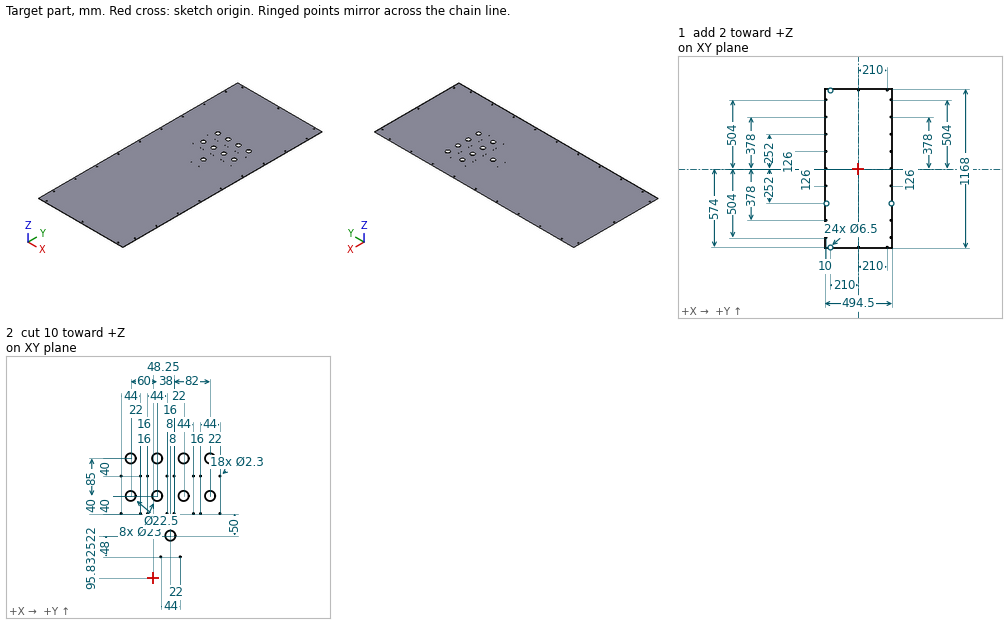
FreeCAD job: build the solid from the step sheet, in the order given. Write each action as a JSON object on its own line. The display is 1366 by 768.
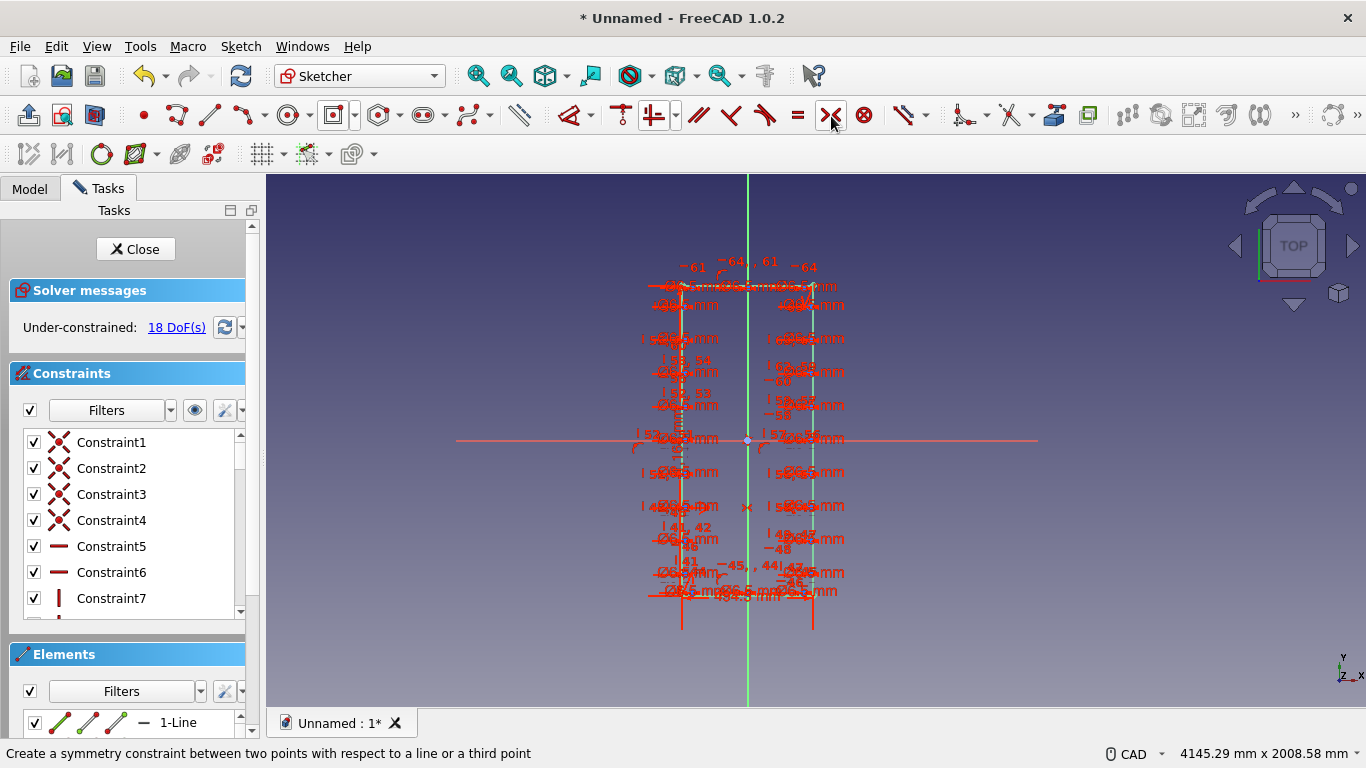
{"action": "left_click", "coordinate": [692, 593]}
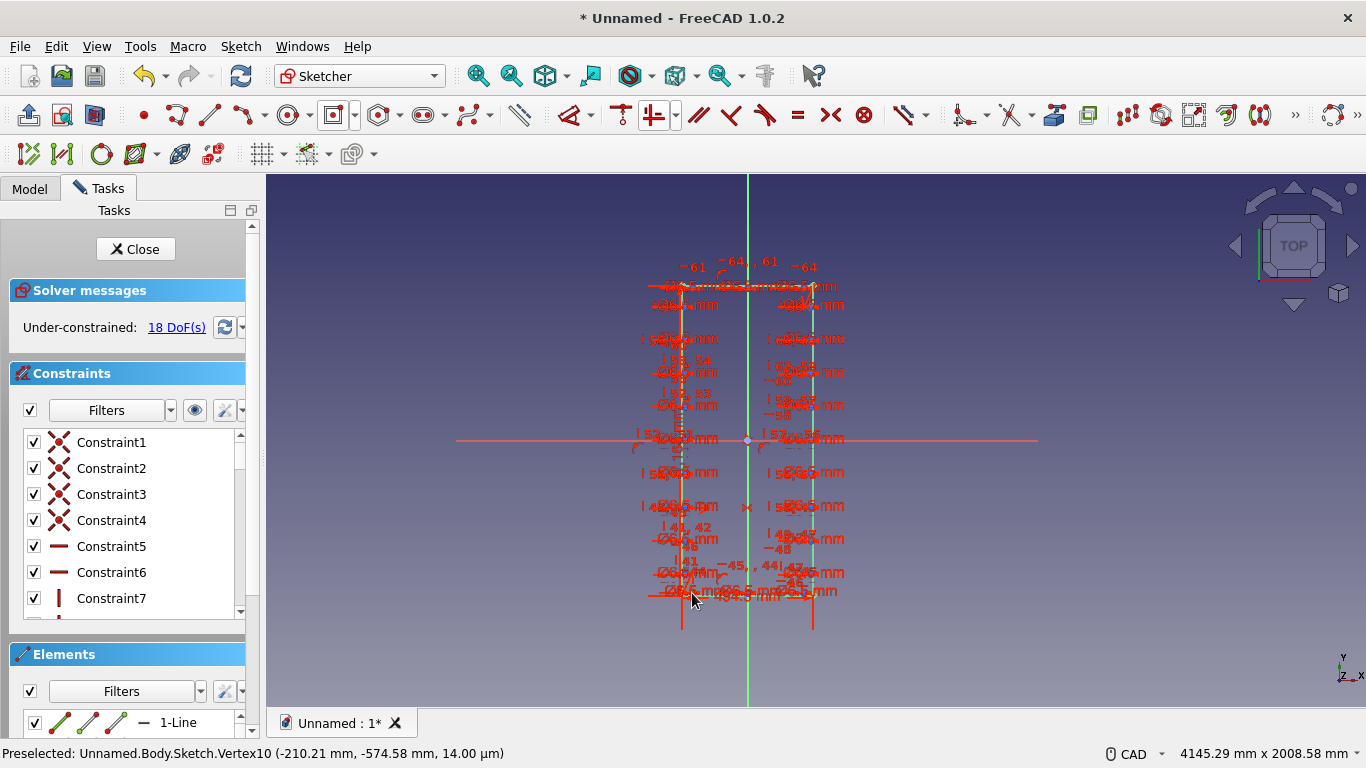
{"action": "left_click", "coordinate": [692, 288]}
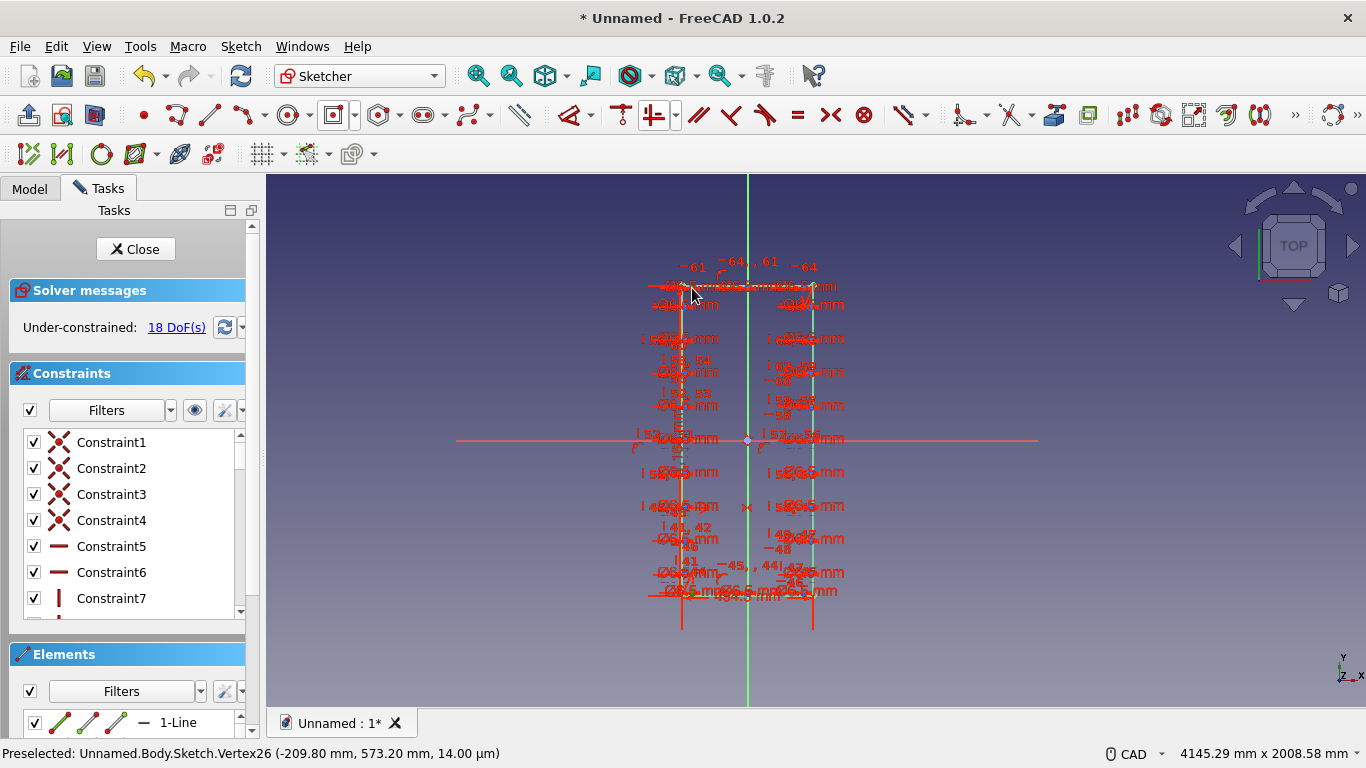
{"action": "left_click", "coordinate": [488, 441]}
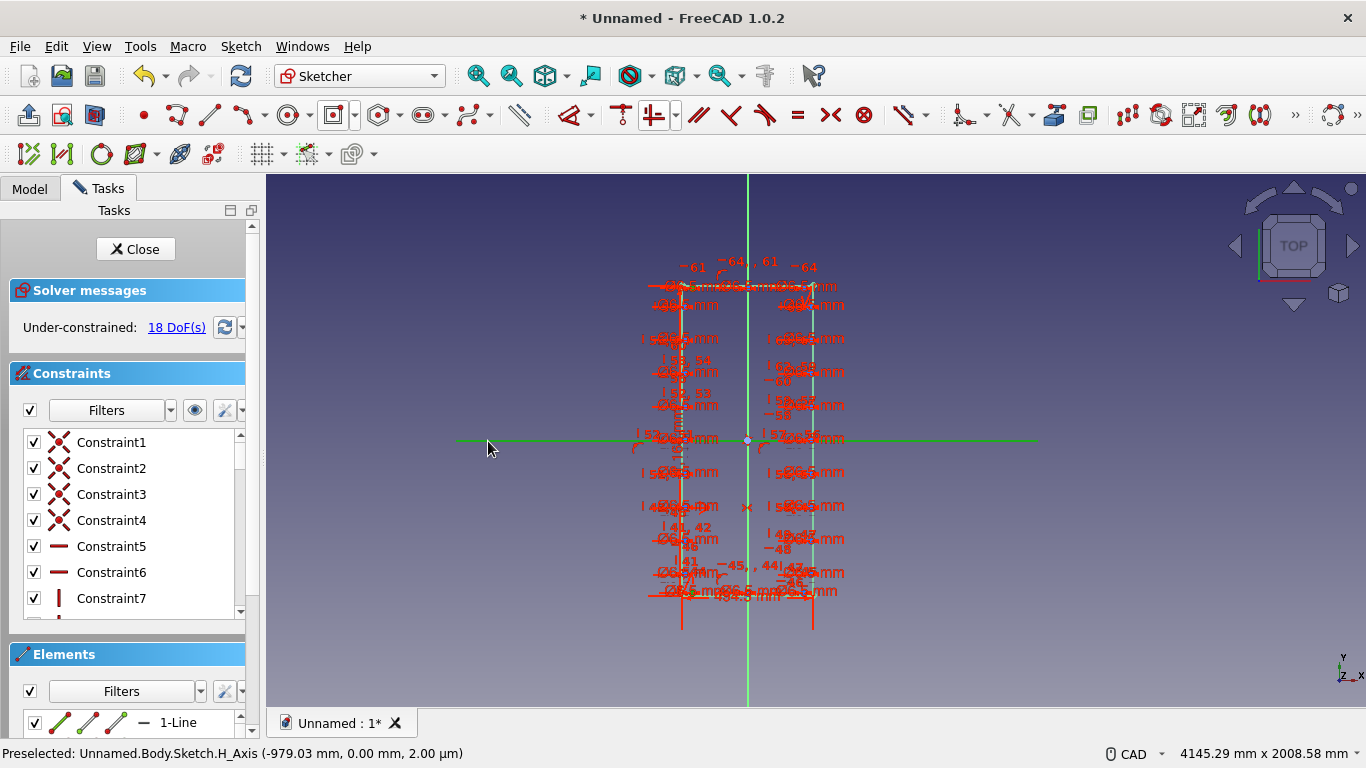
{"action": "left_click", "coordinate": [831, 116]}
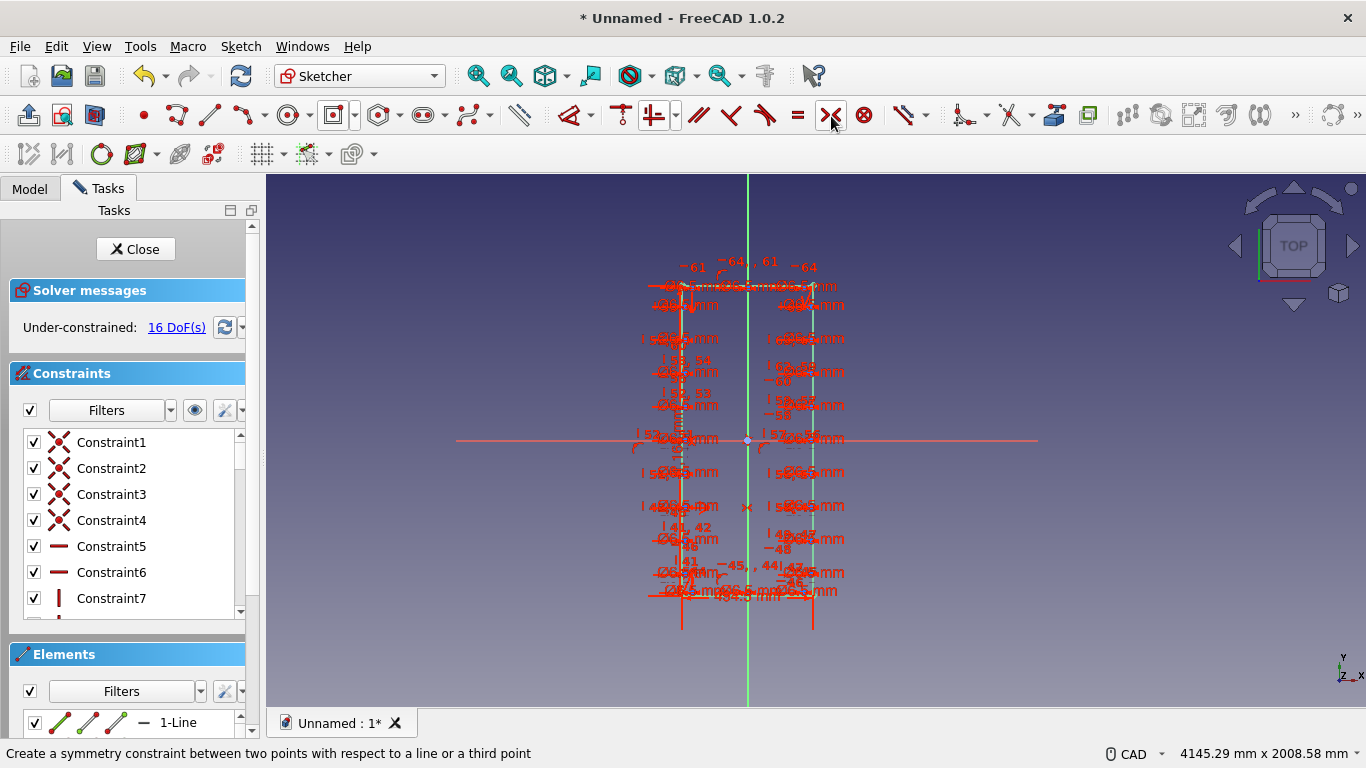
{"action": "left_click", "coordinate": [568, 116]}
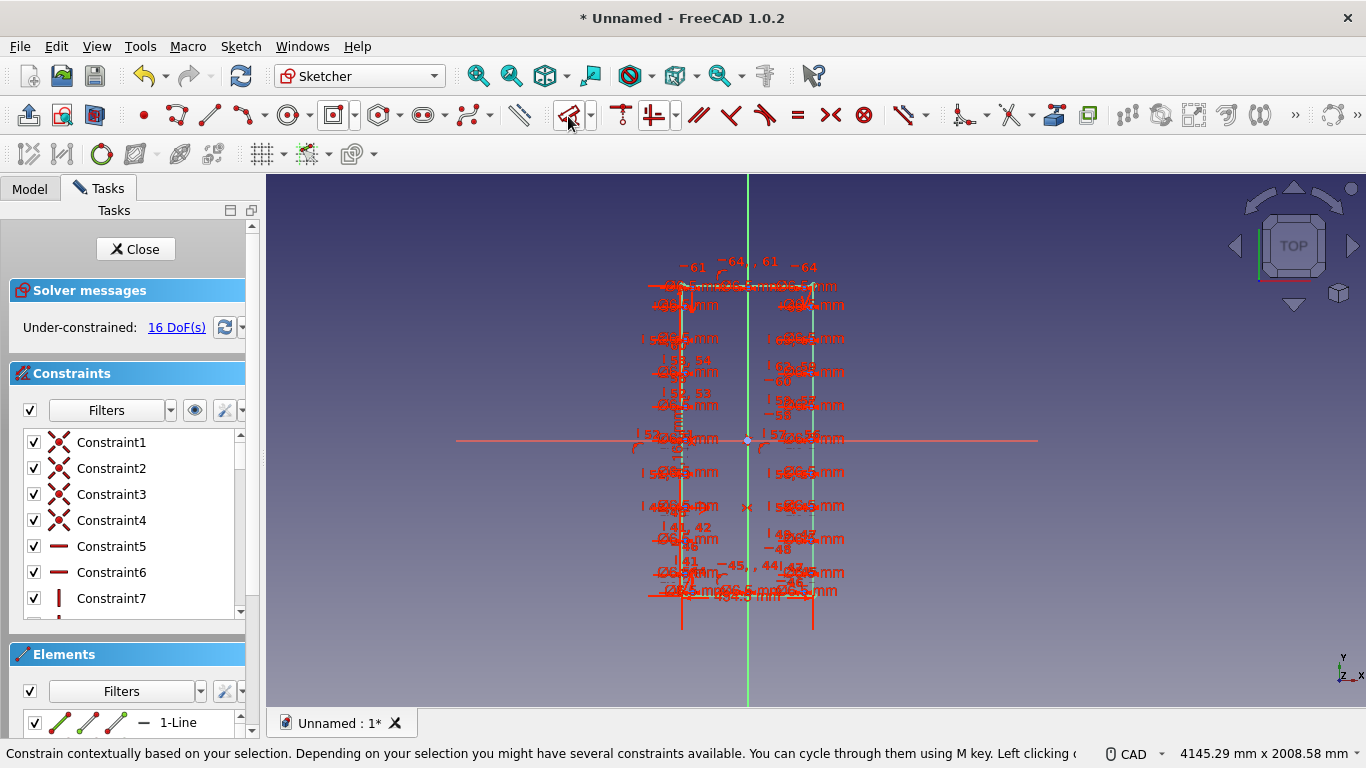
{"action": "left_click", "coordinate": [692, 593]}
{"action": "left_click", "coordinate": [720, 627]}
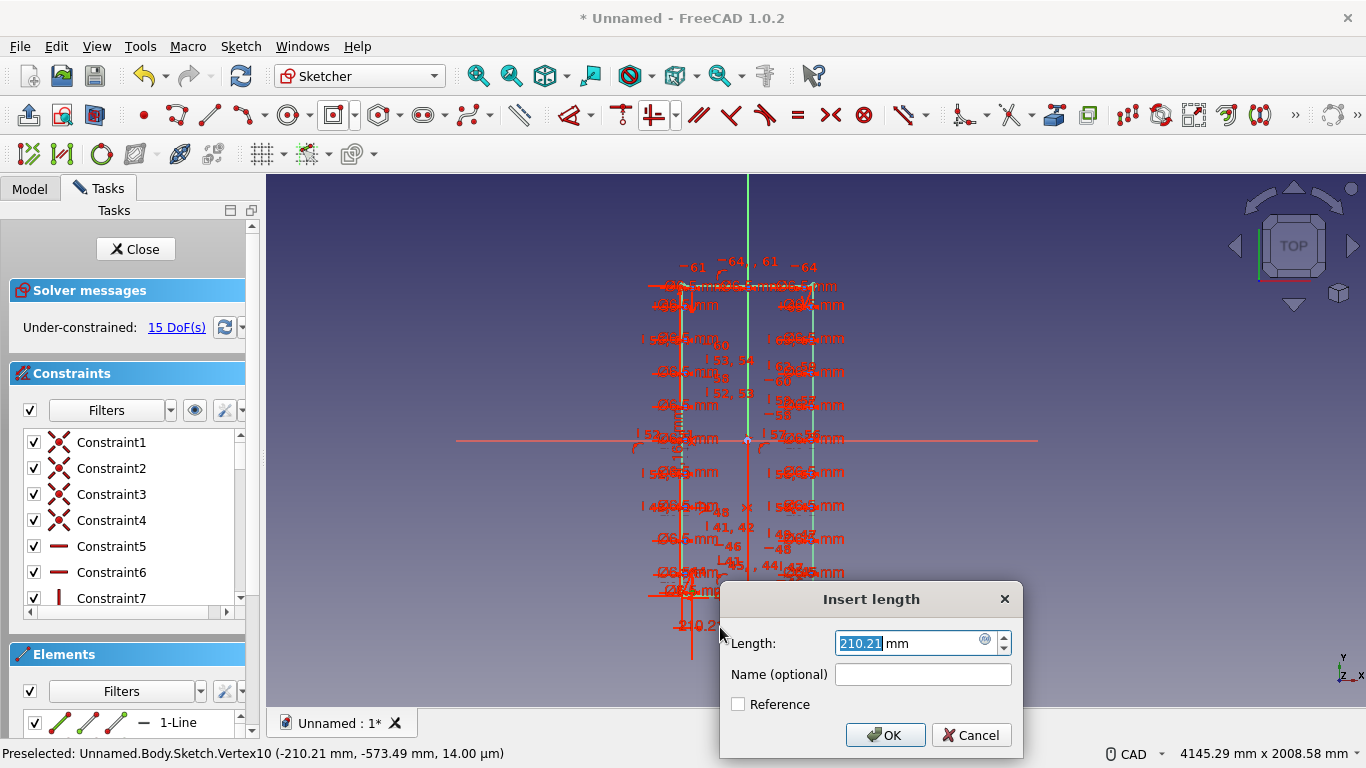
{"action": "type", "text": "210"}
{"action": "key", "text": "Return"}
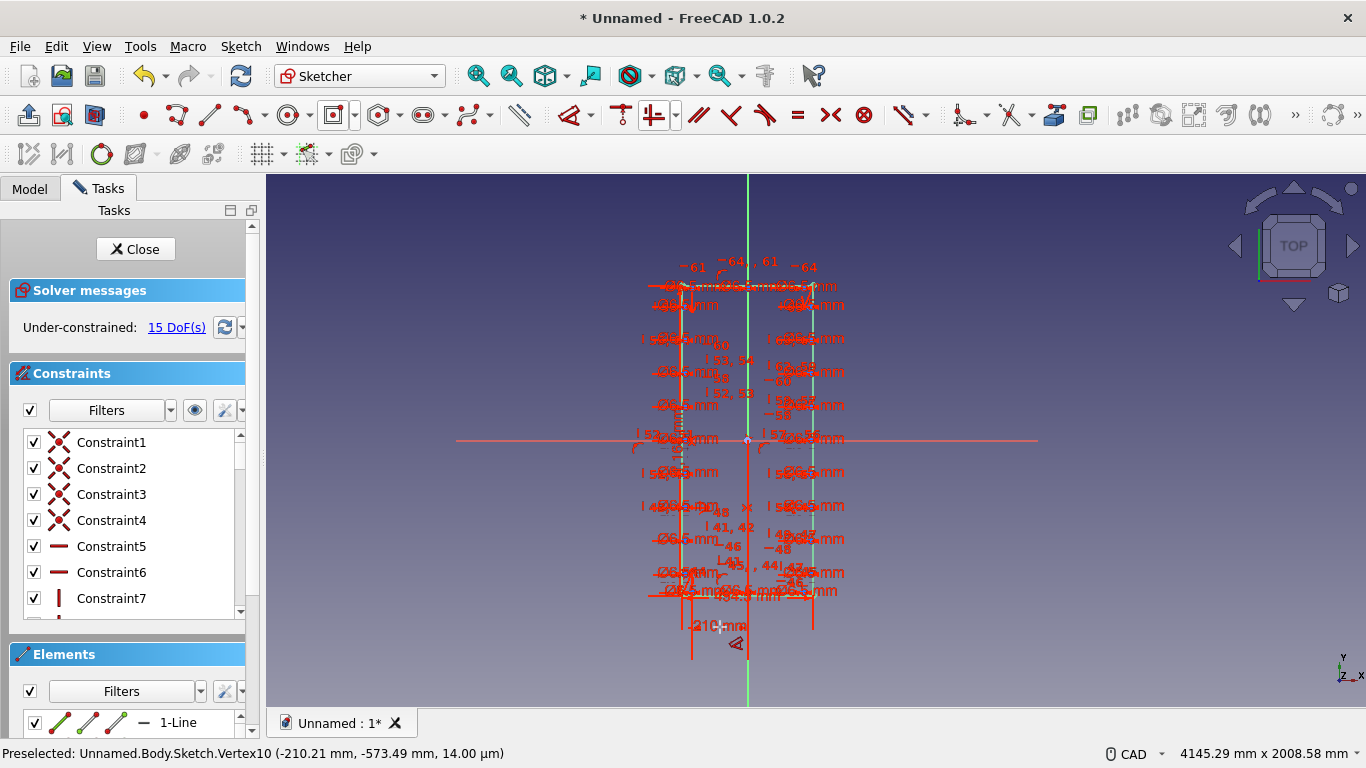
{"action": "left_click", "coordinate": [692, 593]}
{"action": "left_click", "coordinate": [658, 517]}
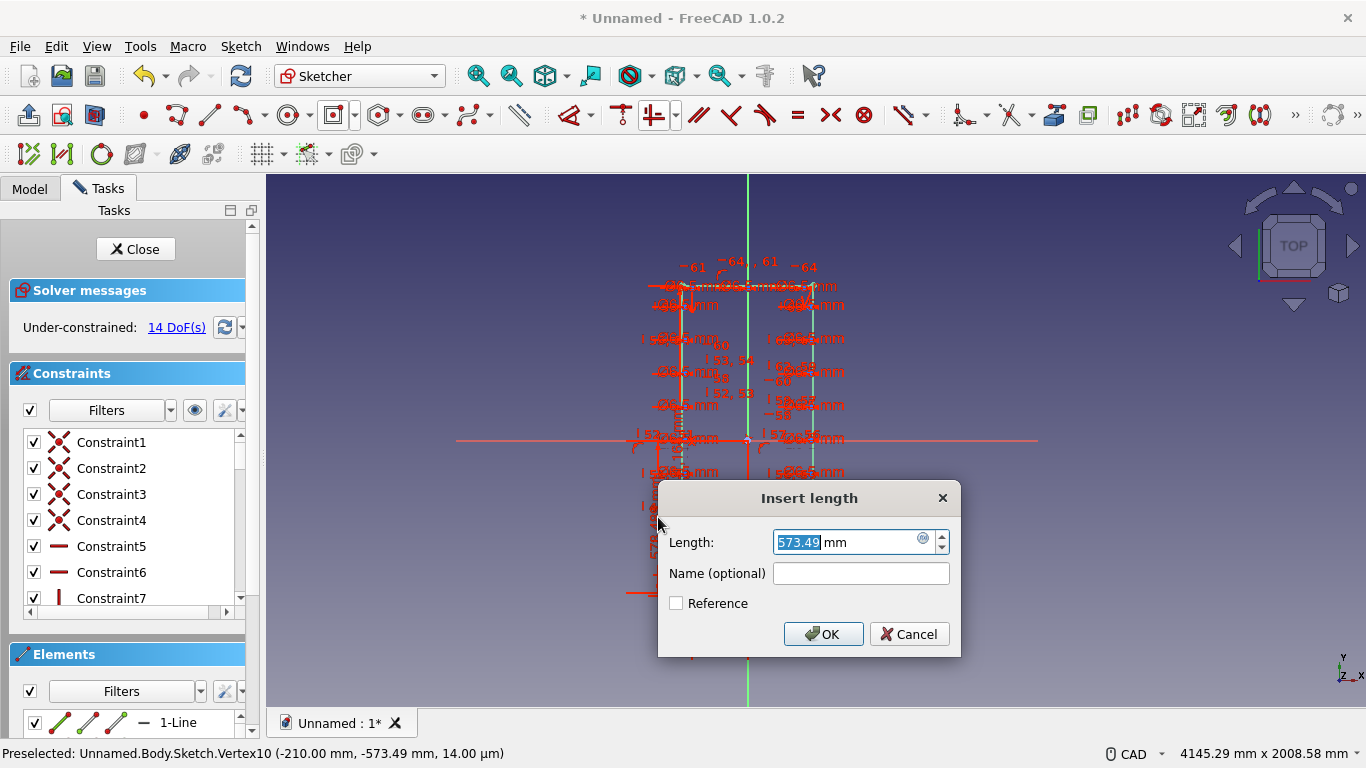
{"action": "type", "text": "574"}
{"action": "key", "text": "Return"}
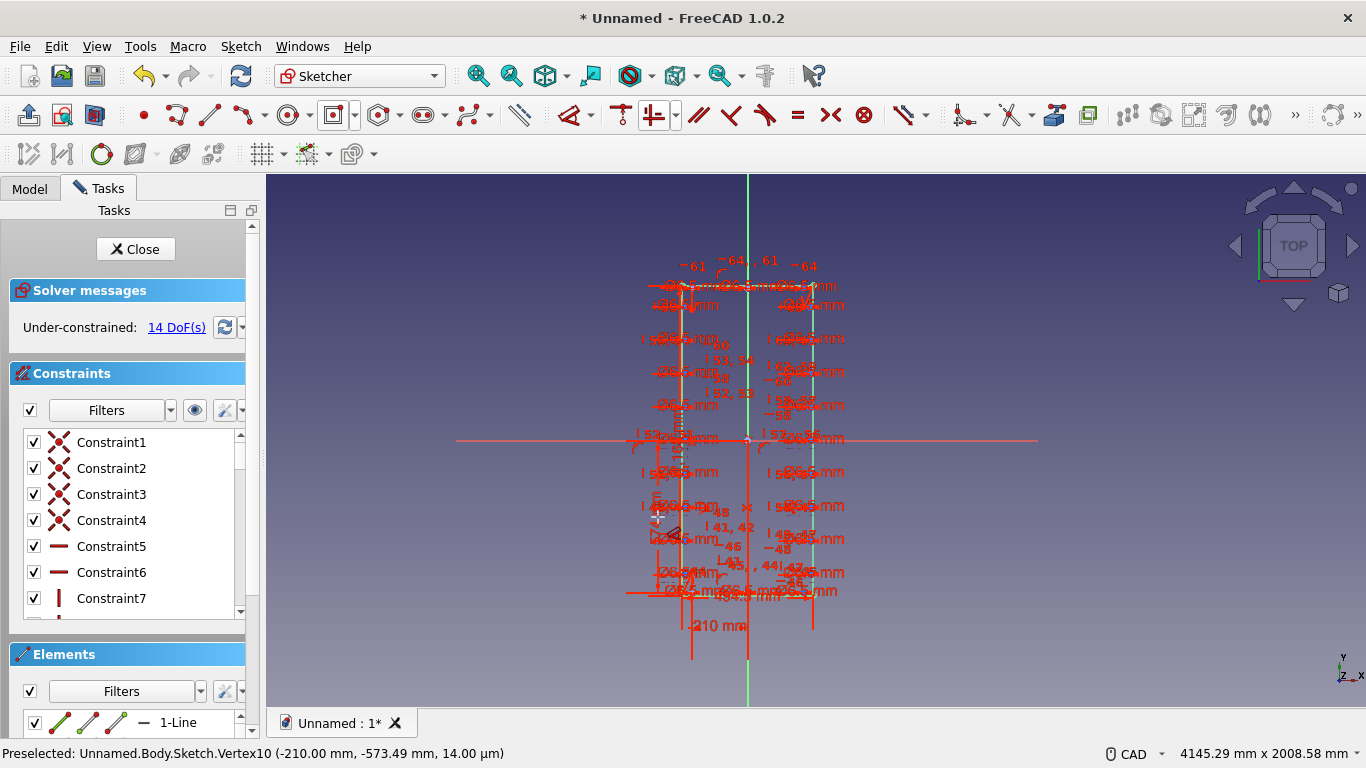
{"action": "left_click", "coordinate": [685, 575]}
{"action": "left_click", "coordinate": [651, 477]}